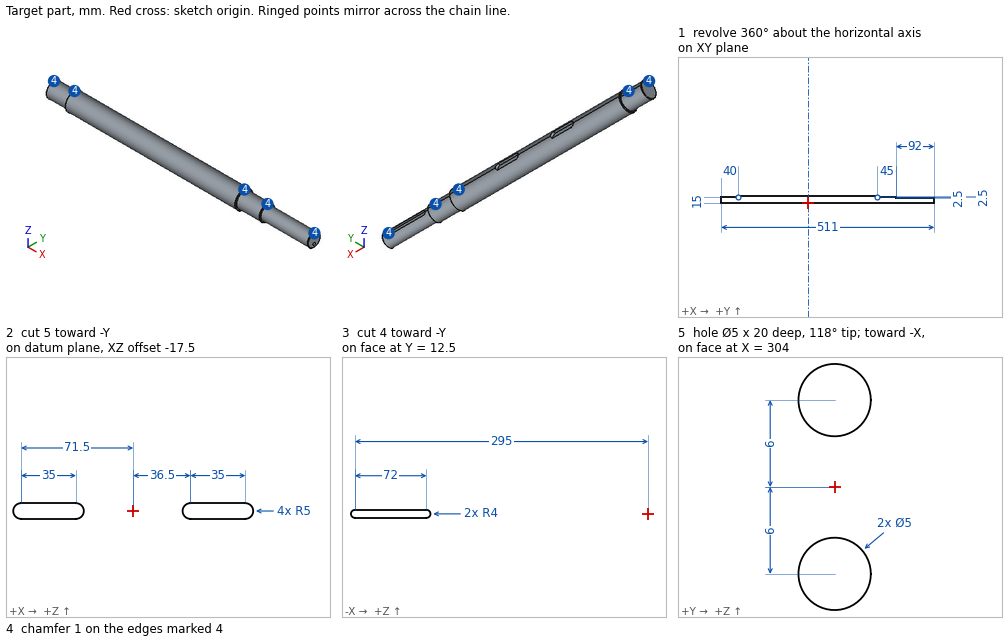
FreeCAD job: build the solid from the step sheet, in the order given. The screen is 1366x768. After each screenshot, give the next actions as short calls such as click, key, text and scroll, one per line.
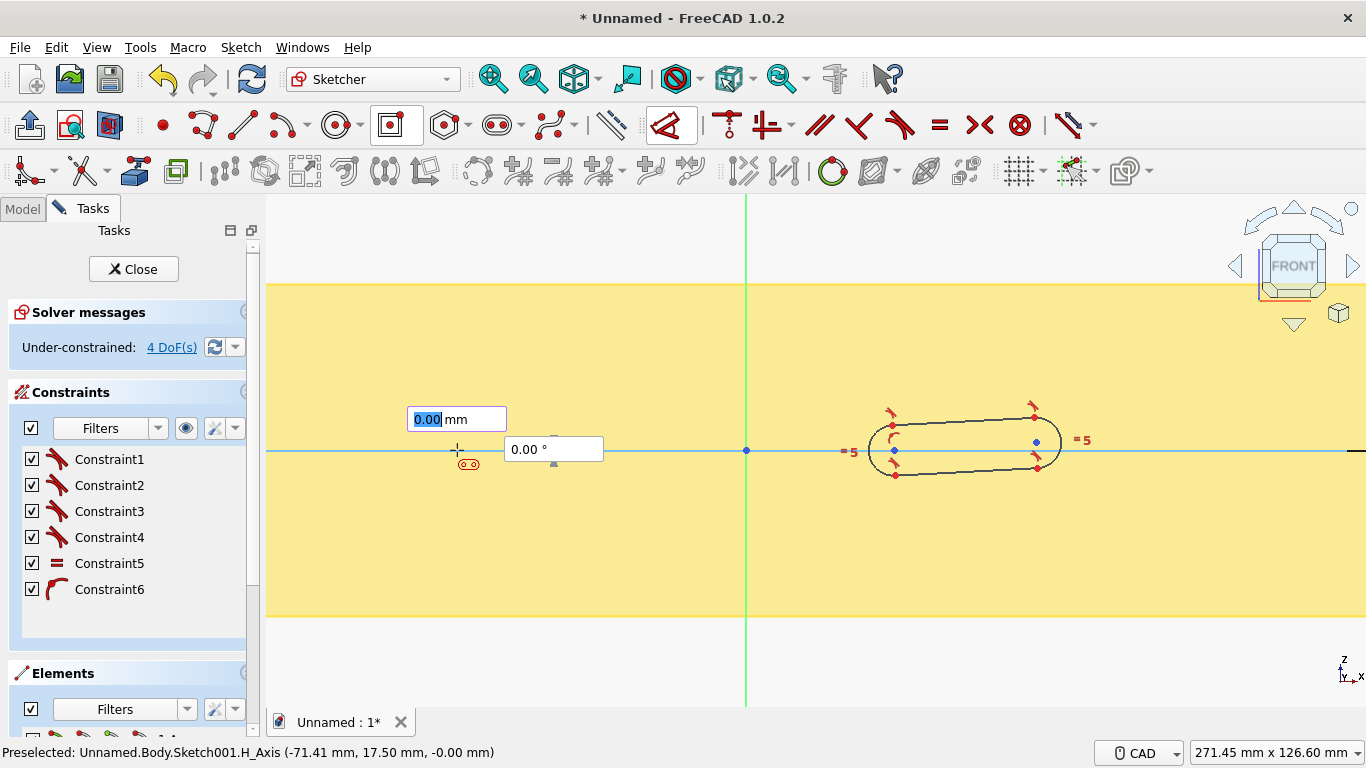
click(598, 442)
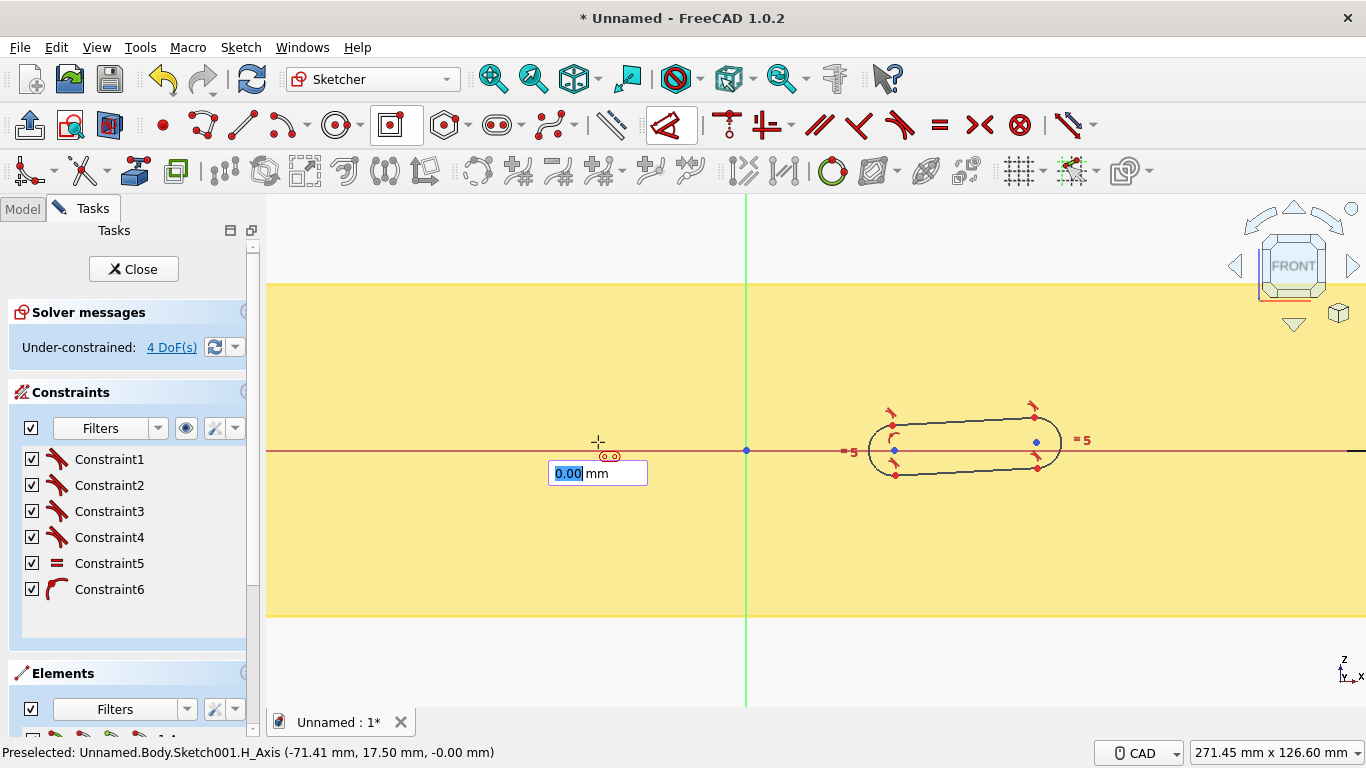
click(528, 471)
key(Escape)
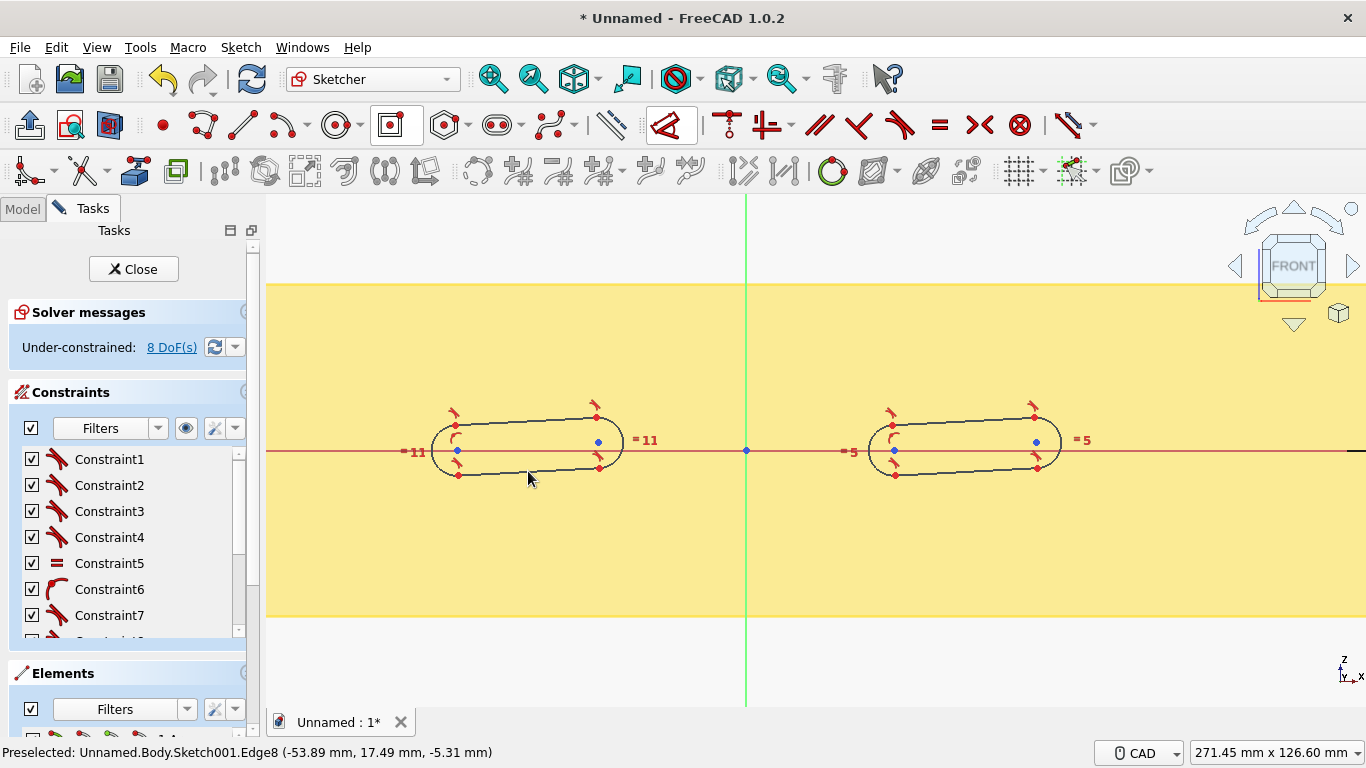
click(935, 423)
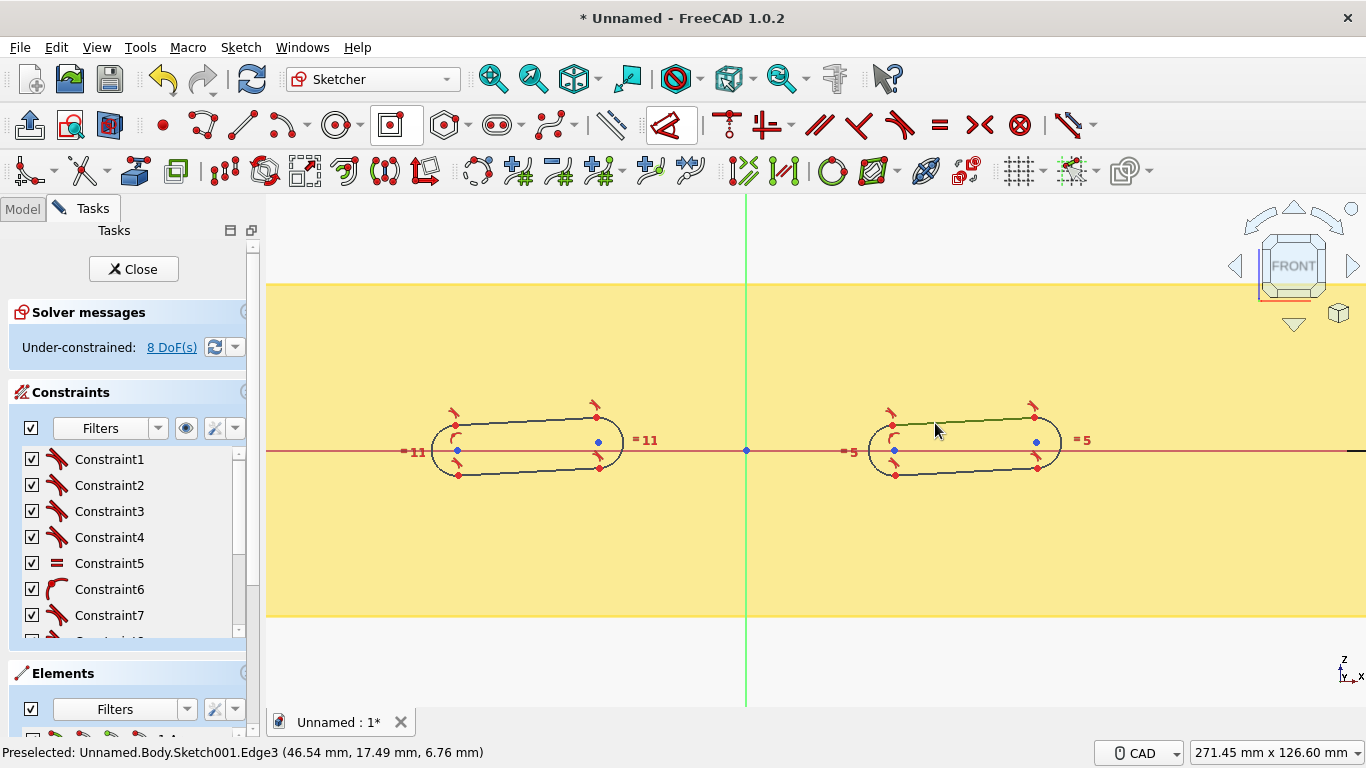
click(794, 126)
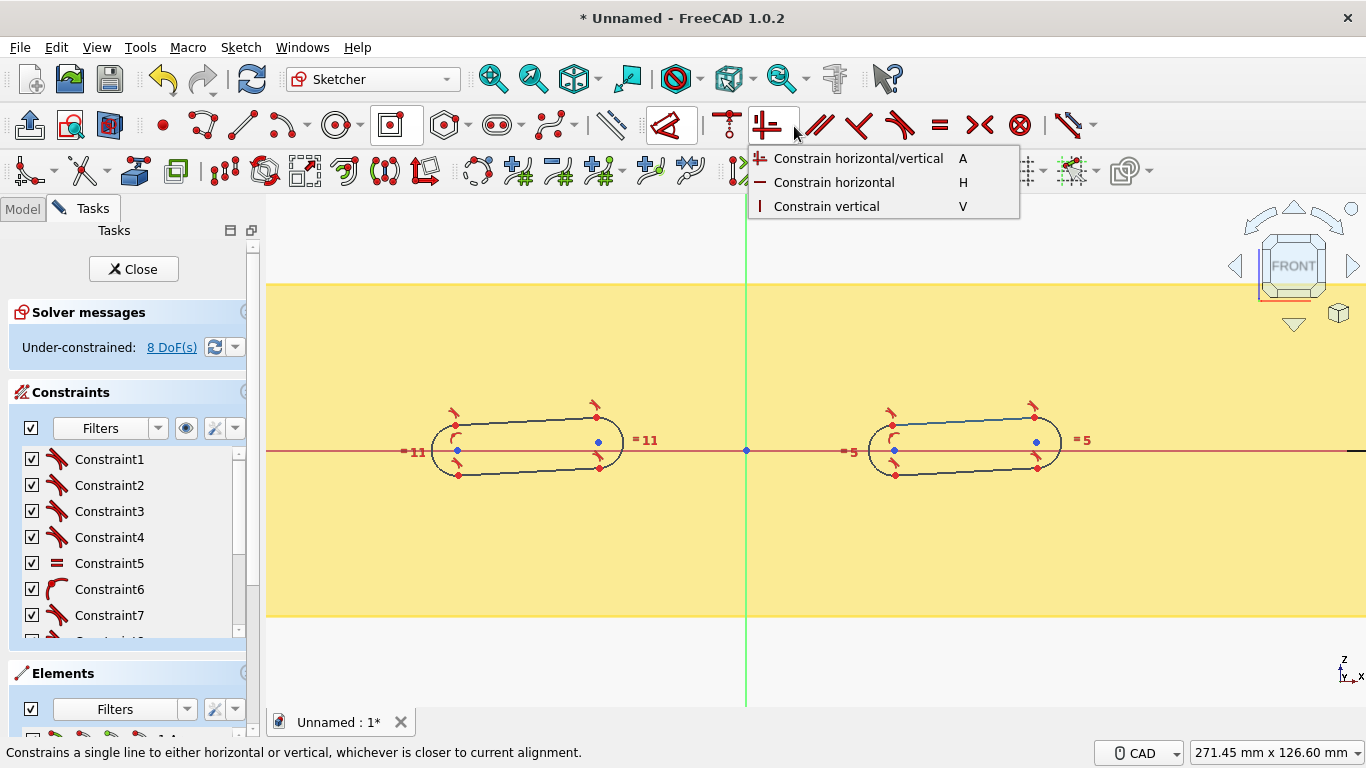
click(884, 182)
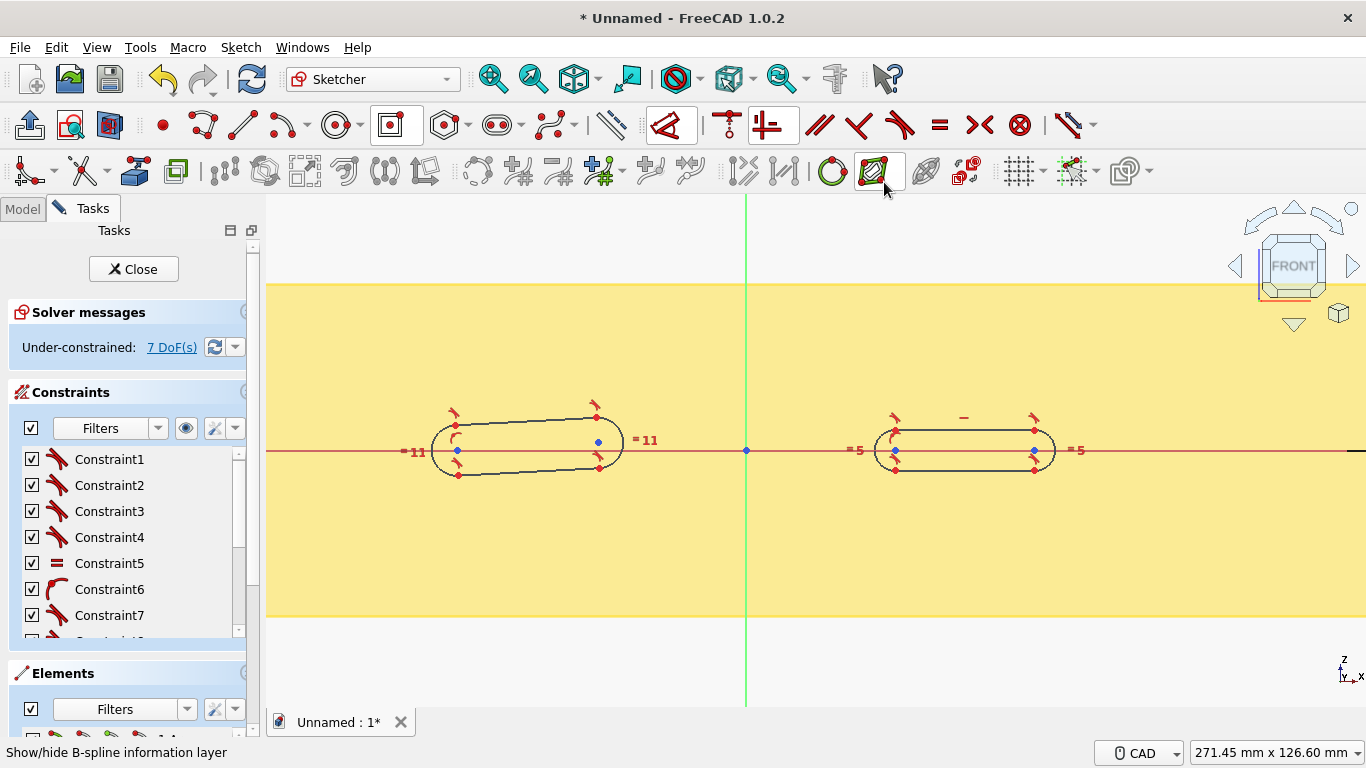
click(498, 423)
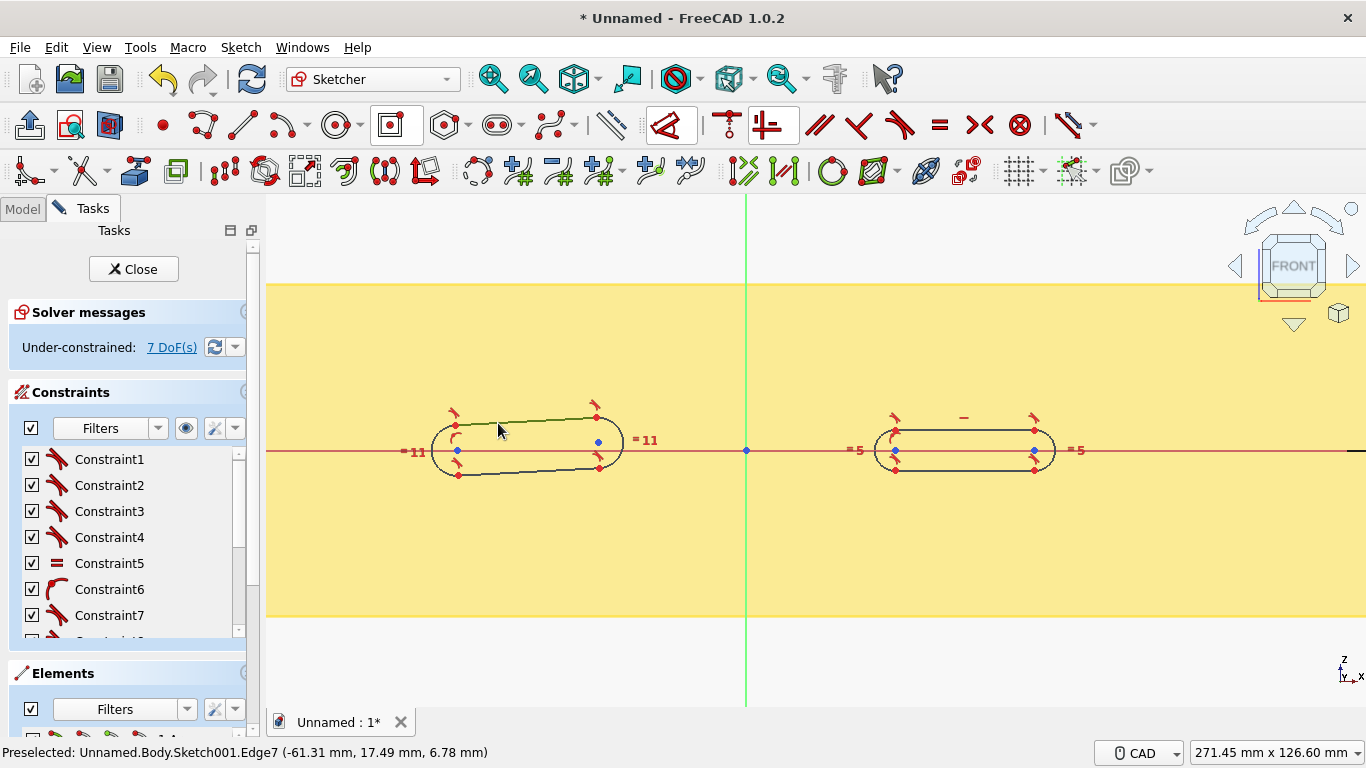
click(794, 126)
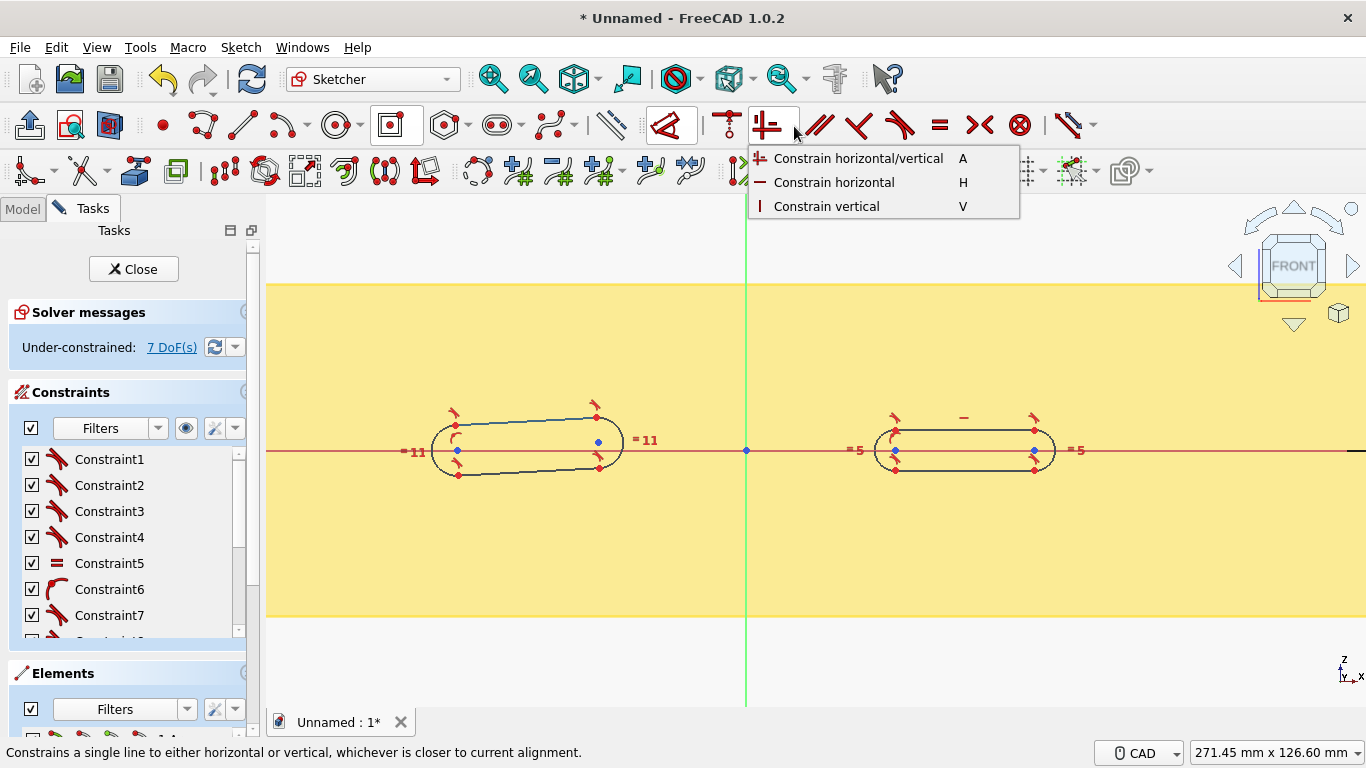
click(884, 182)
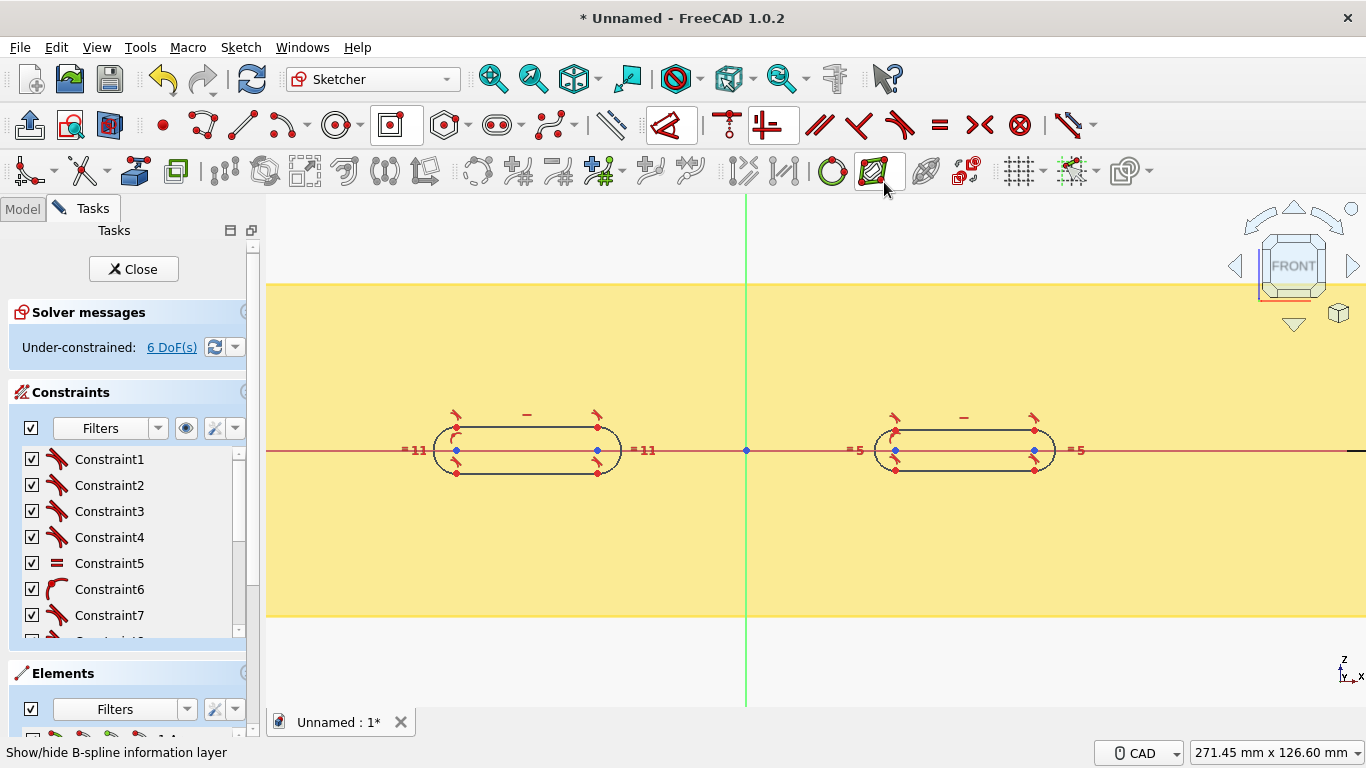
click(879, 438)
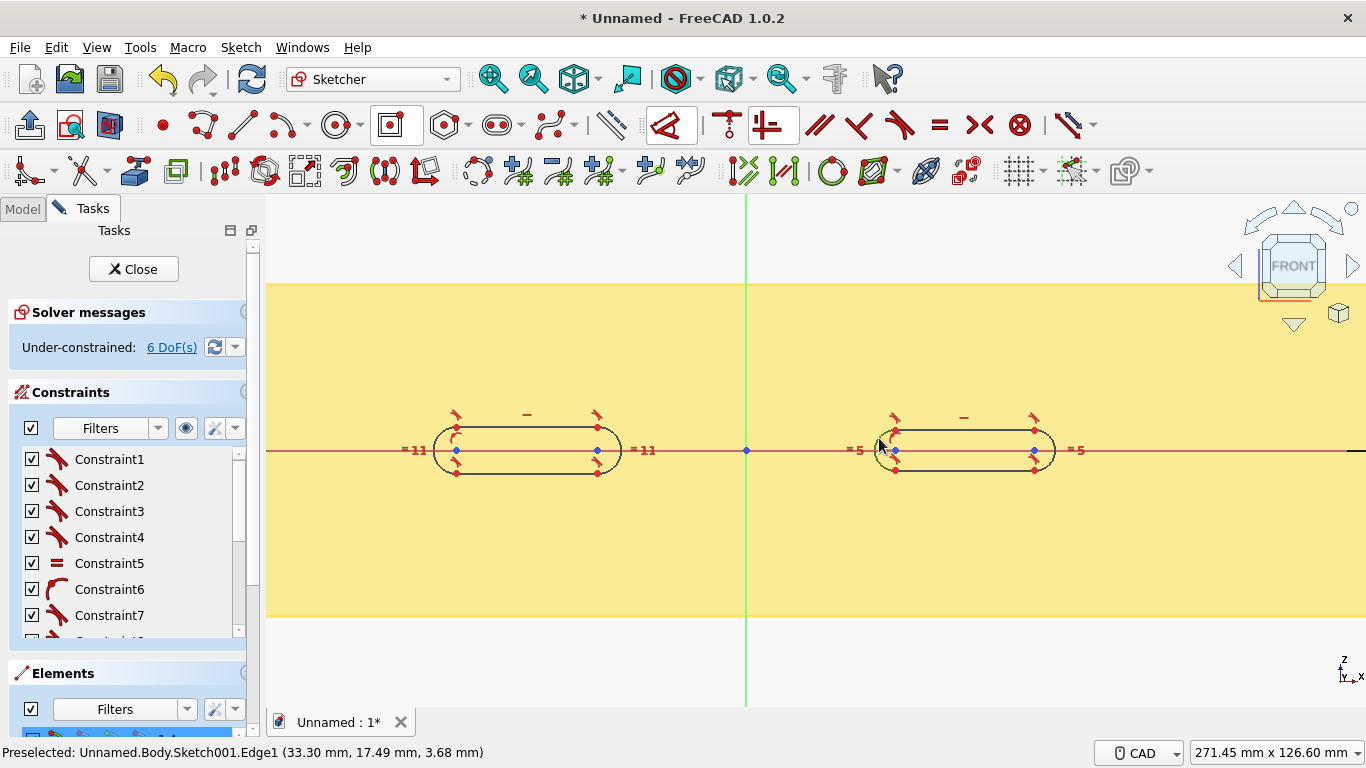
click(438, 437)